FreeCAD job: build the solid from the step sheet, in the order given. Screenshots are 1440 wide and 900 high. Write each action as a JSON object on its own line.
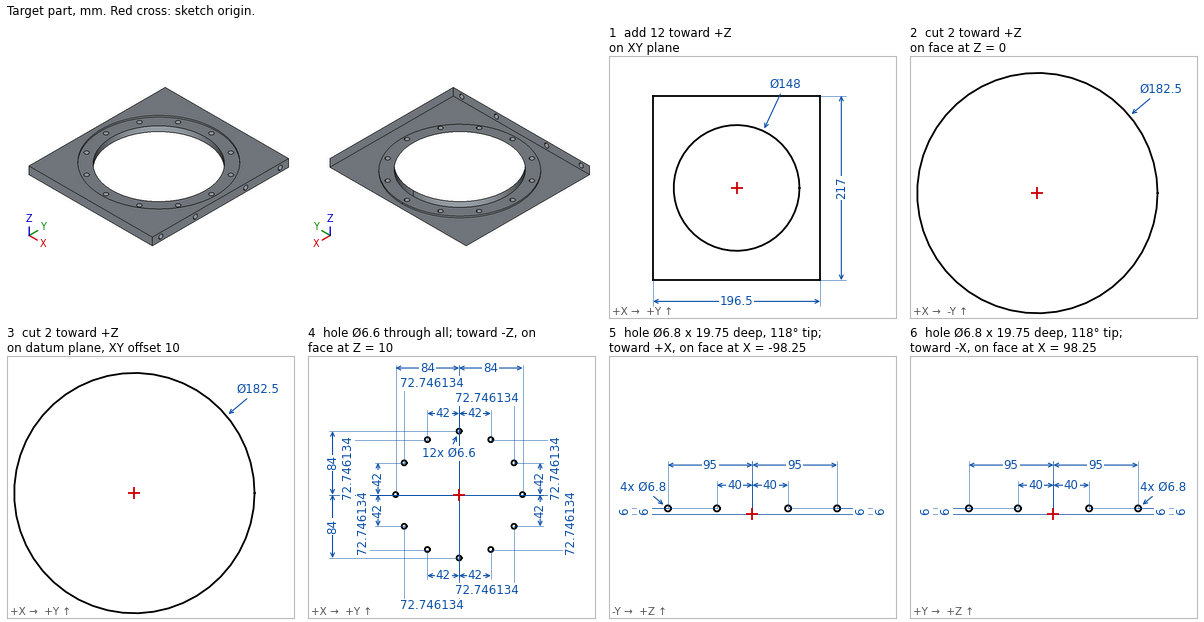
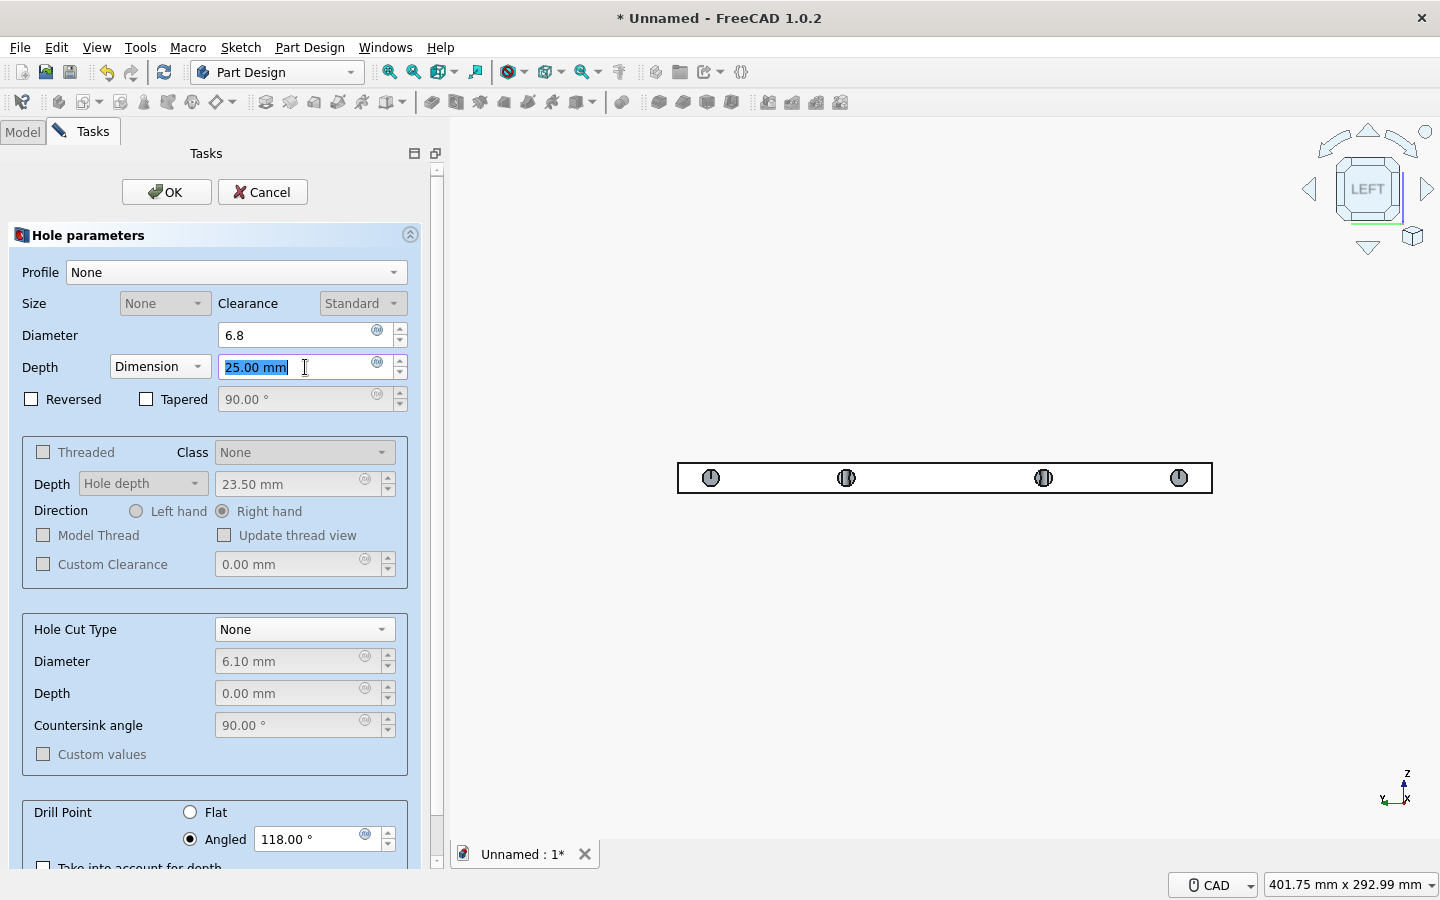
{"action": "type", "text": "19.75"}
{"action": "key", "text": "Tab"}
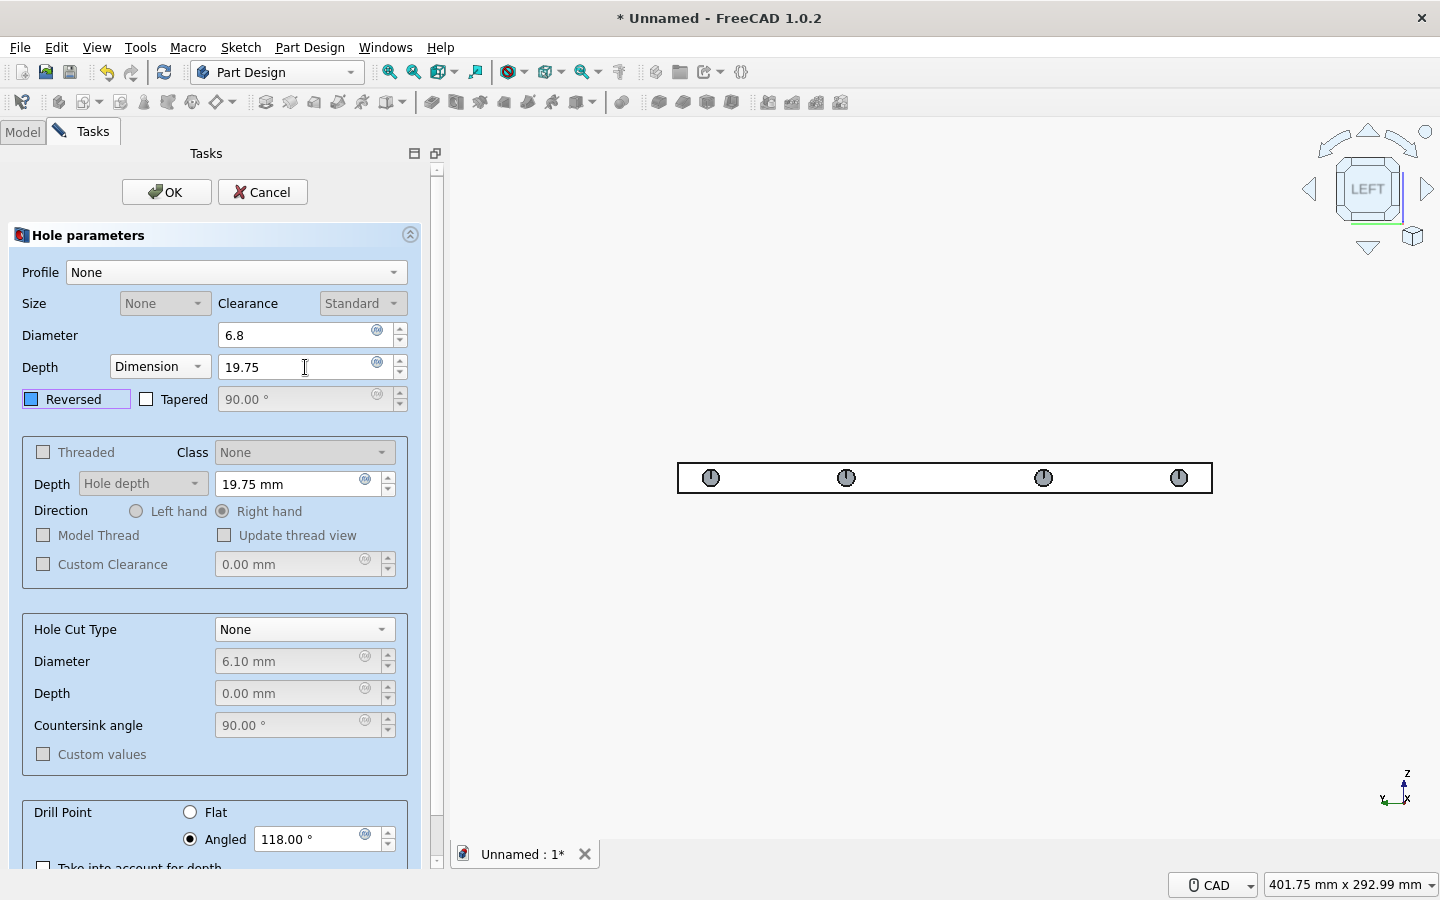
{"action": "left_click", "coordinate": [167, 192]}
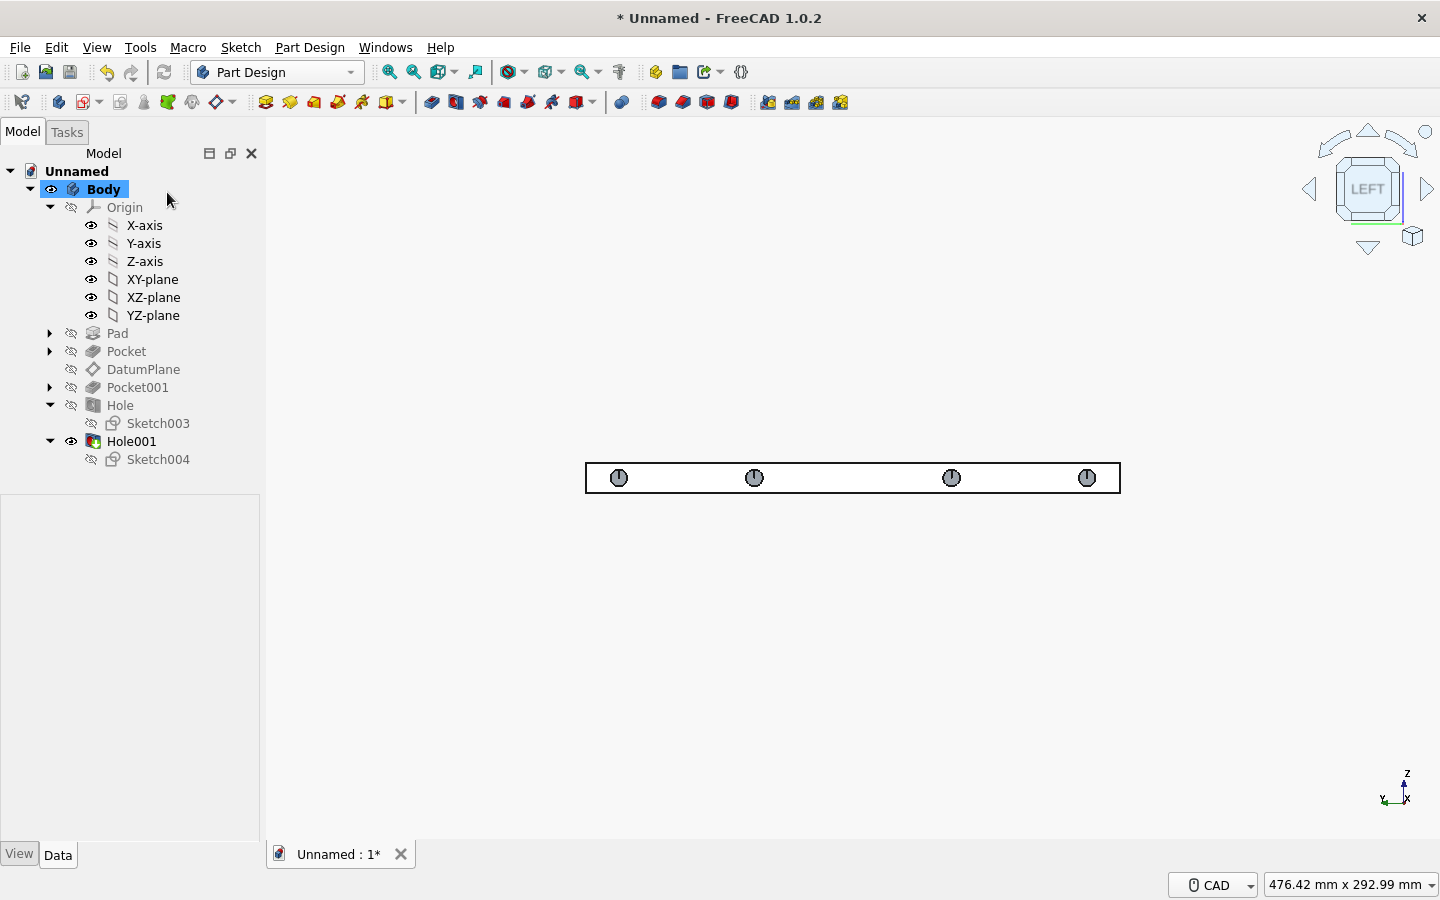
{"action": "key", "text": "0"}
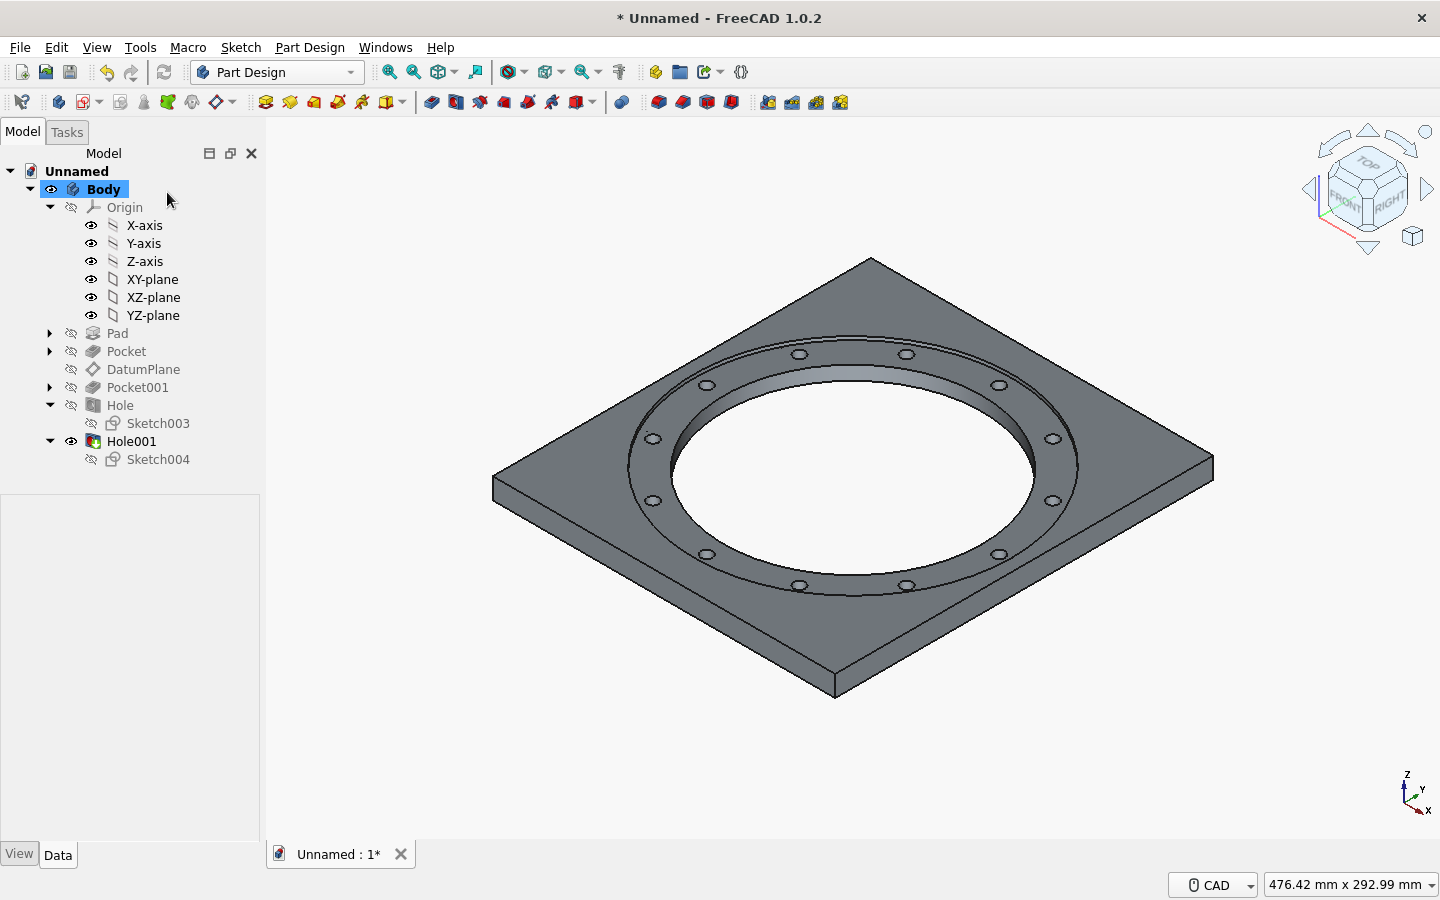
{"action": "left_click", "coordinate": [1186, 482]}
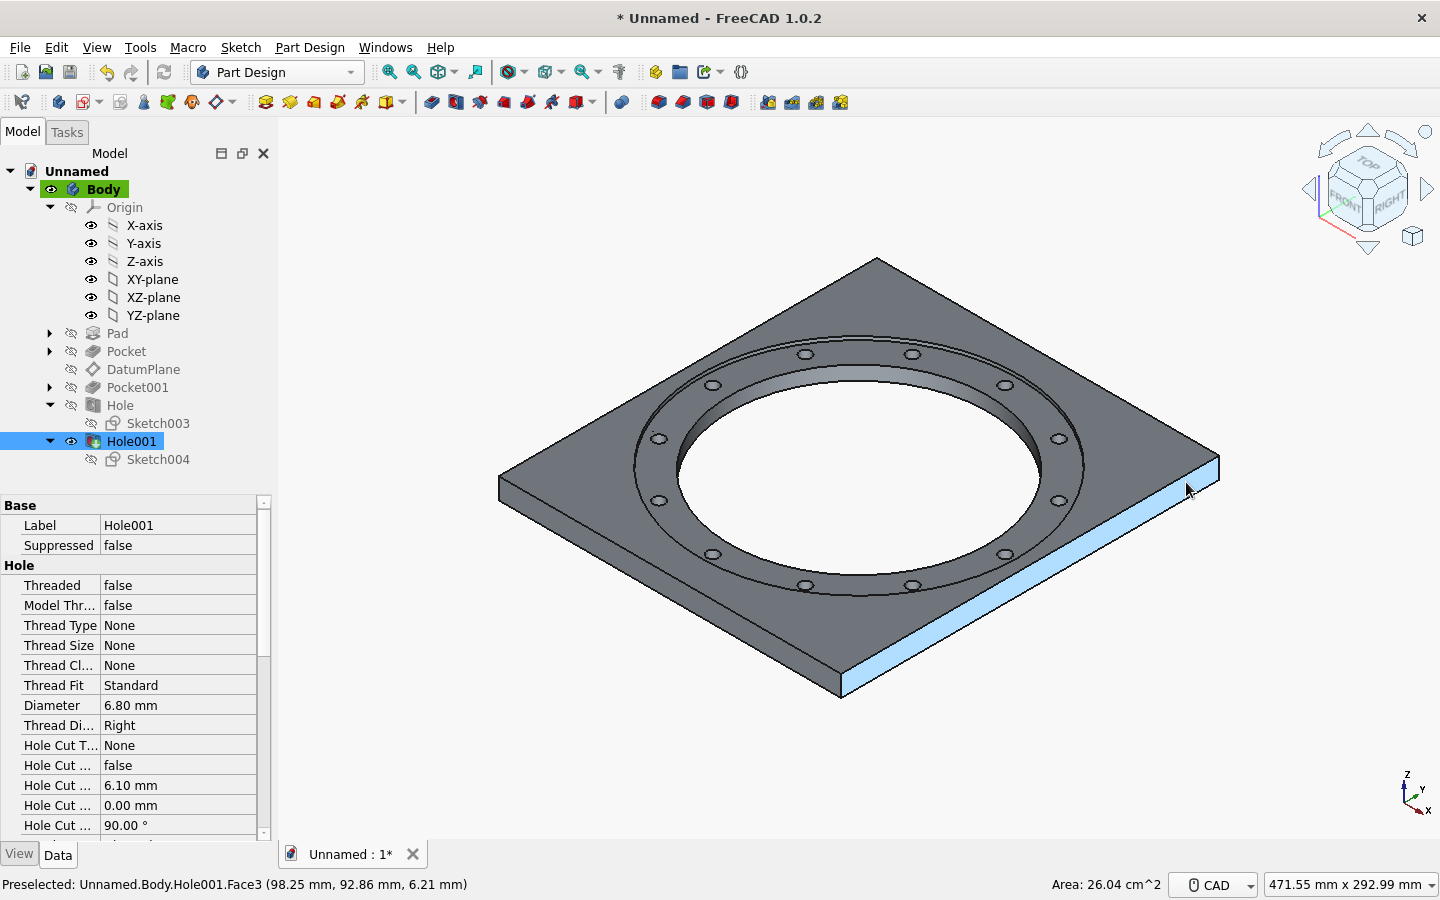
{"action": "left_click", "coordinate": [84, 102]}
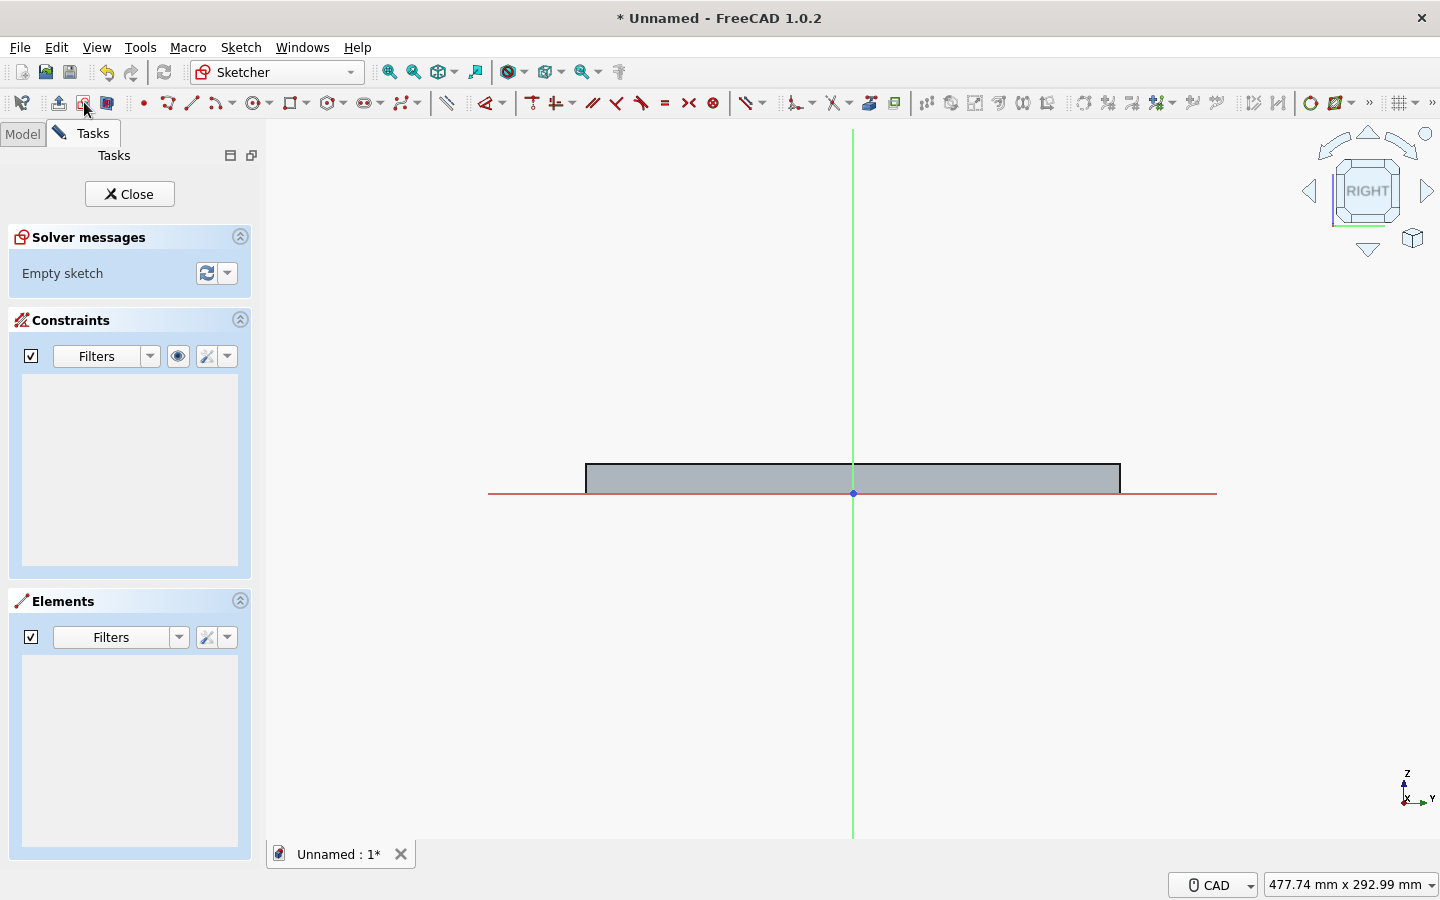
{"action": "scroll", "coordinate": [992, 489], "scroll_direction": "up", "scroll_amount": 2}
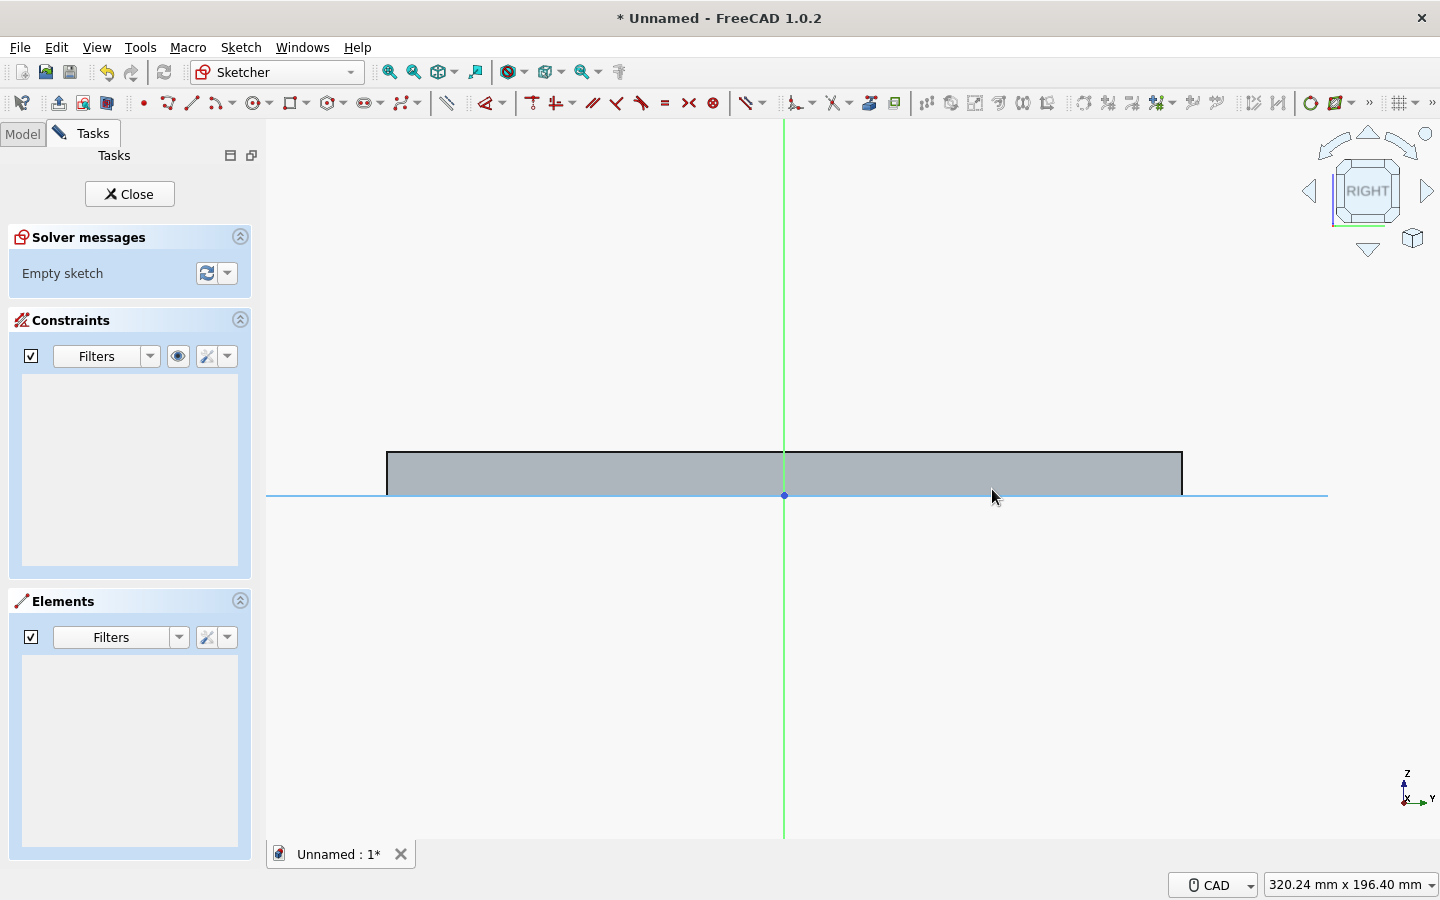
{"action": "left_click", "coordinate": [254, 104]}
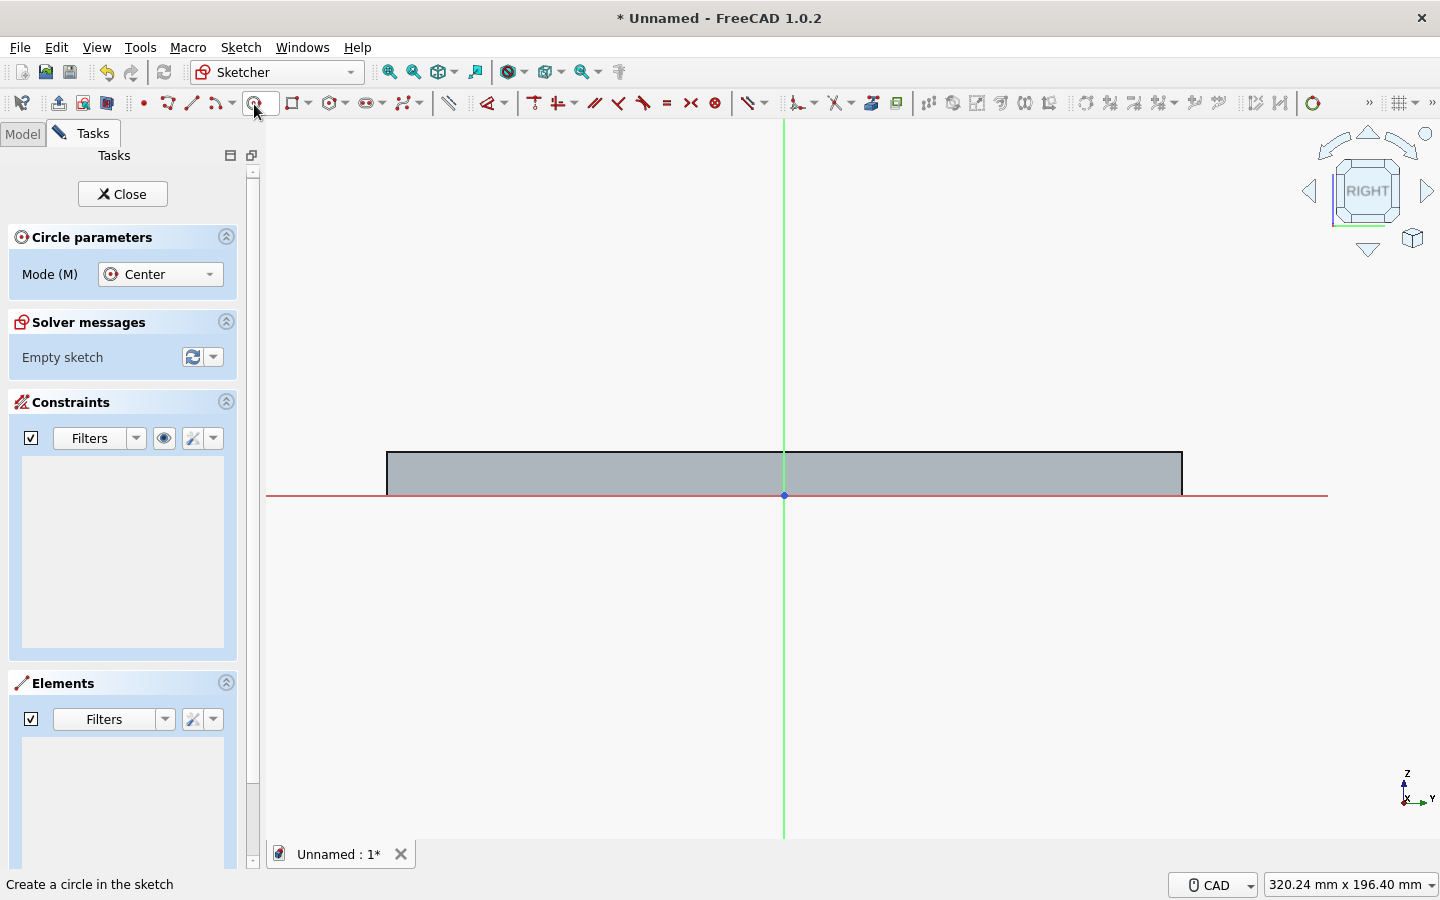
{"action": "scroll", "coordinate": [1133, 474], "scroll_direction": "up", "scroll_amount": 3}